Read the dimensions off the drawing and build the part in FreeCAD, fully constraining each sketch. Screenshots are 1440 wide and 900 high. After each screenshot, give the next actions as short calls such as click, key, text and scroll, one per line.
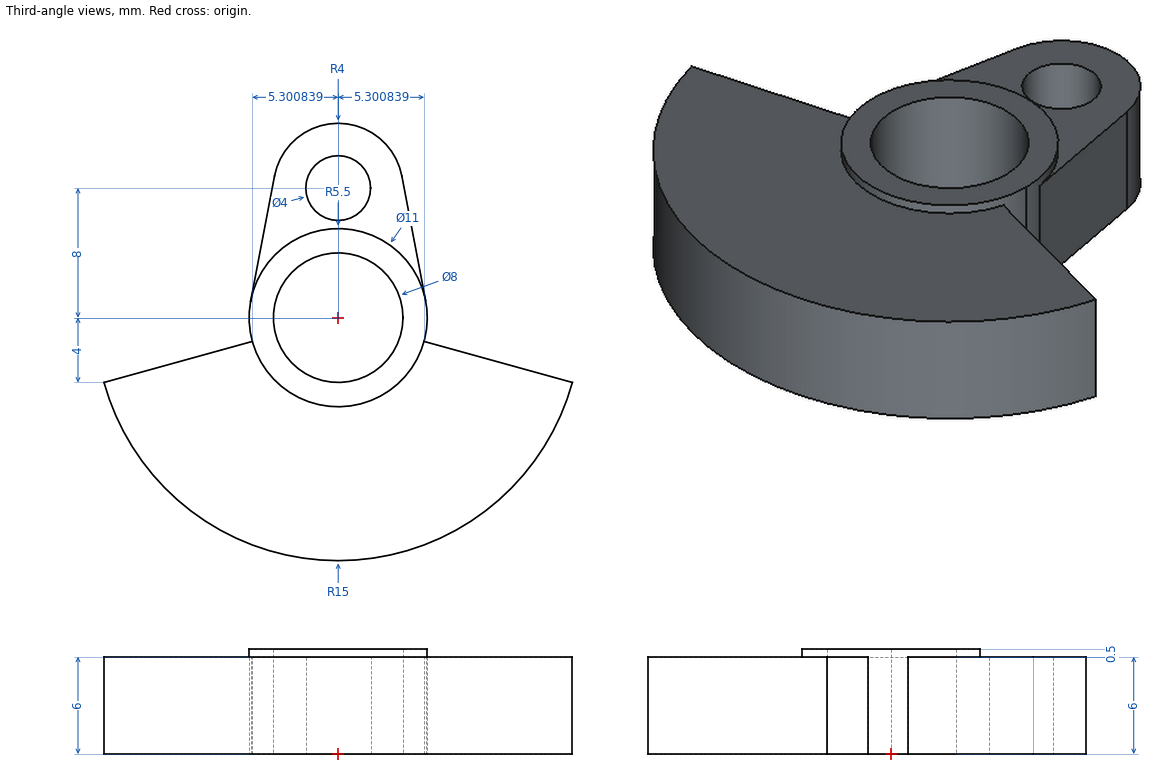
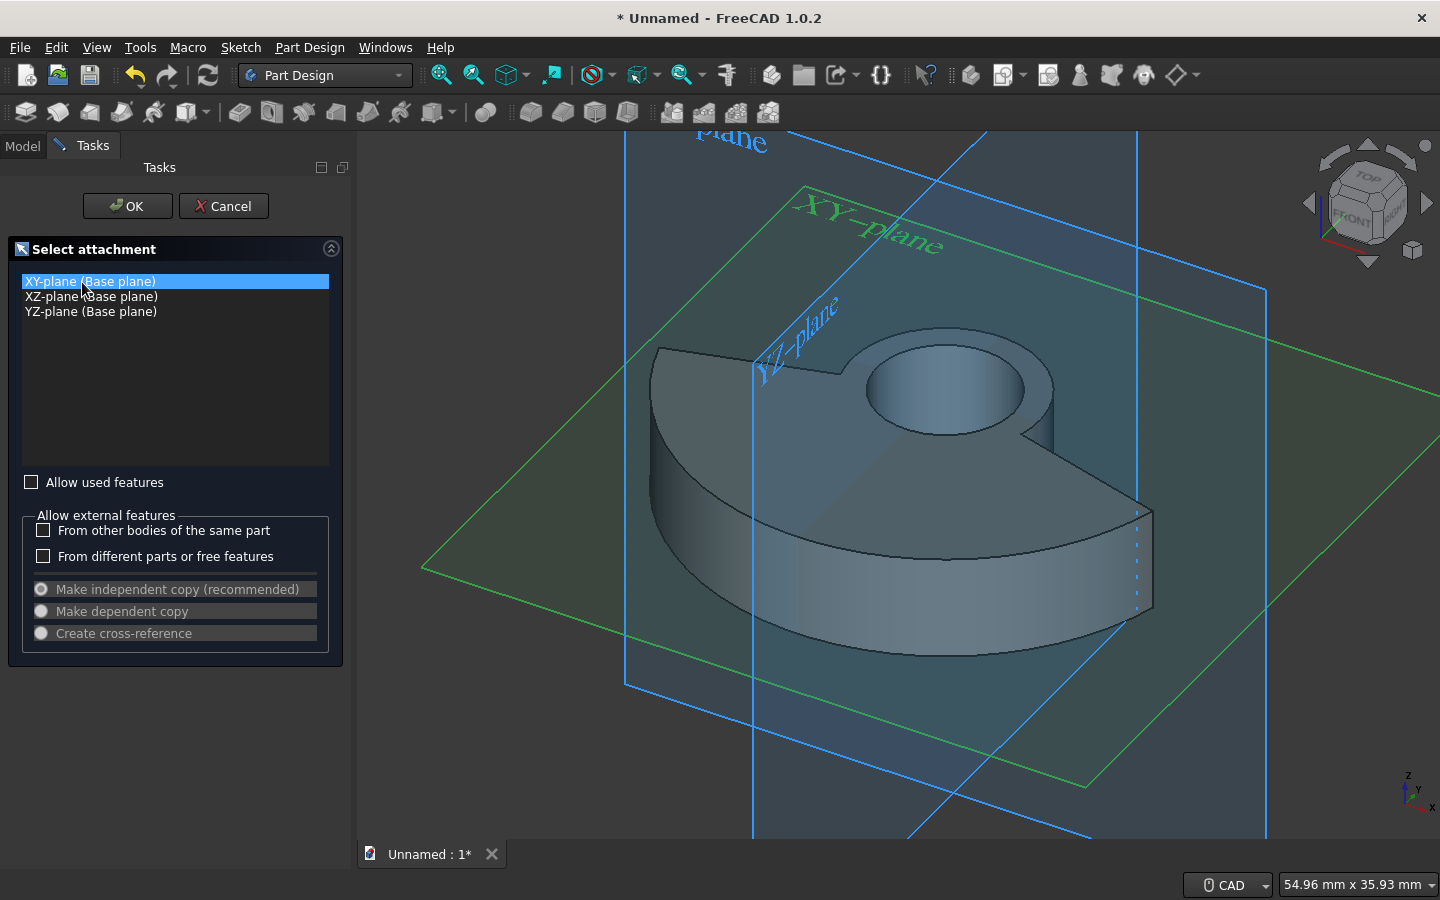
click(128, 206)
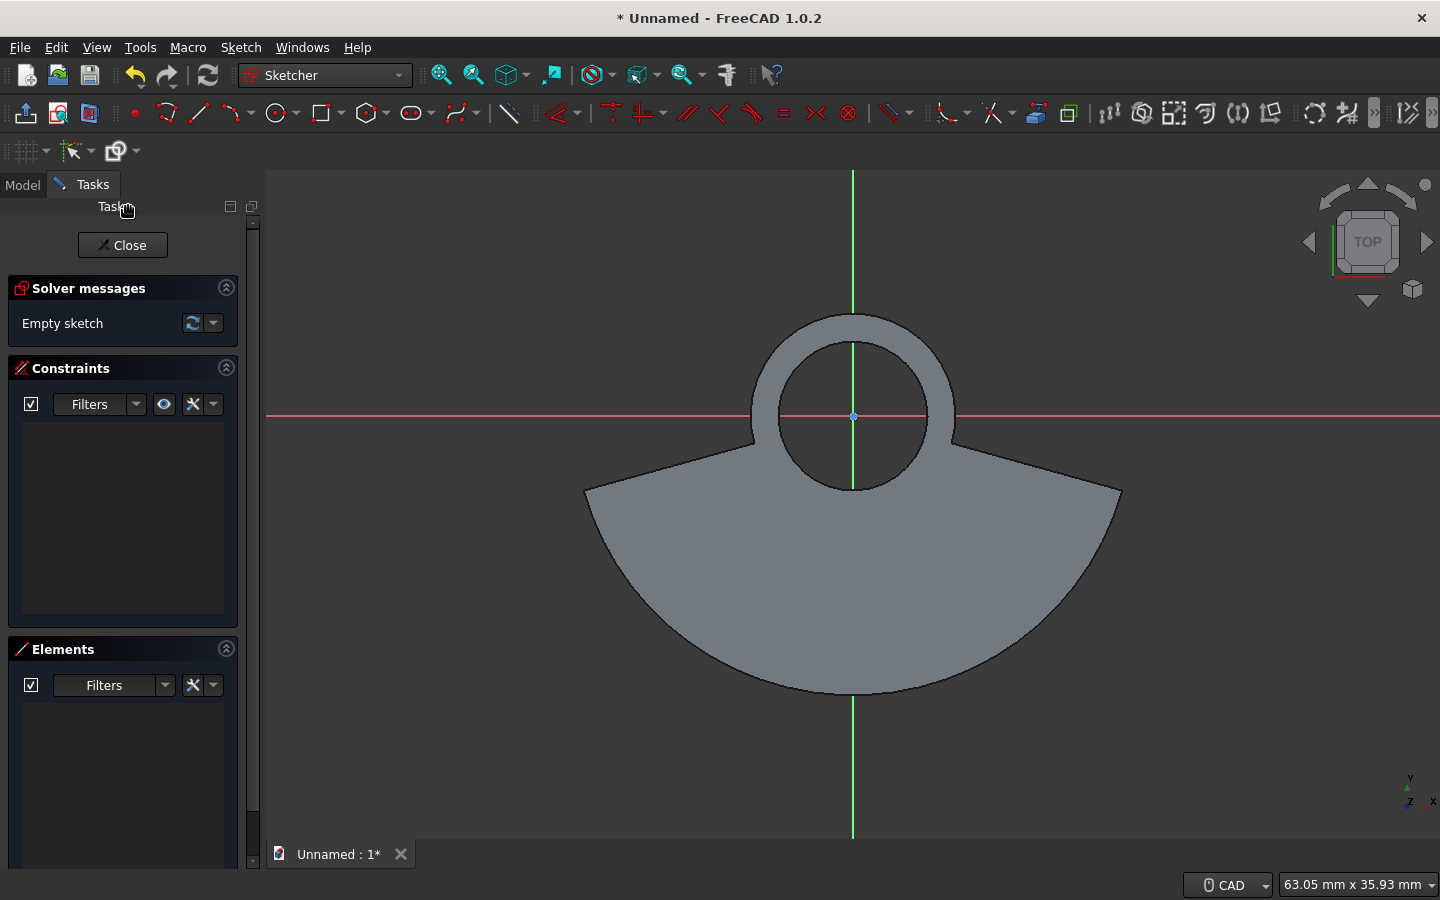
key(q)
key(s)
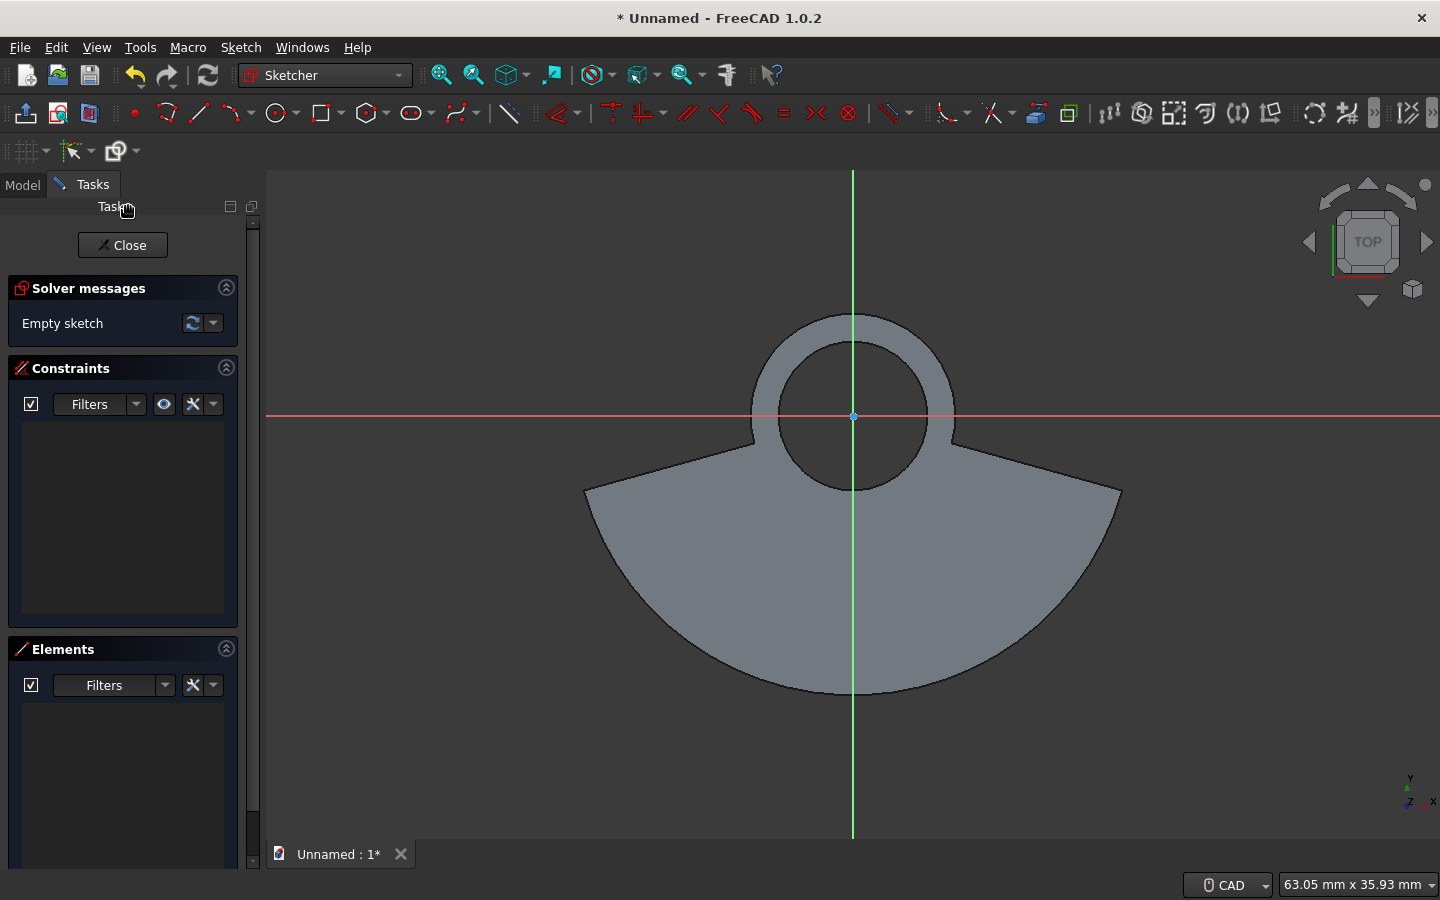
scroll(784, 504, down, 5)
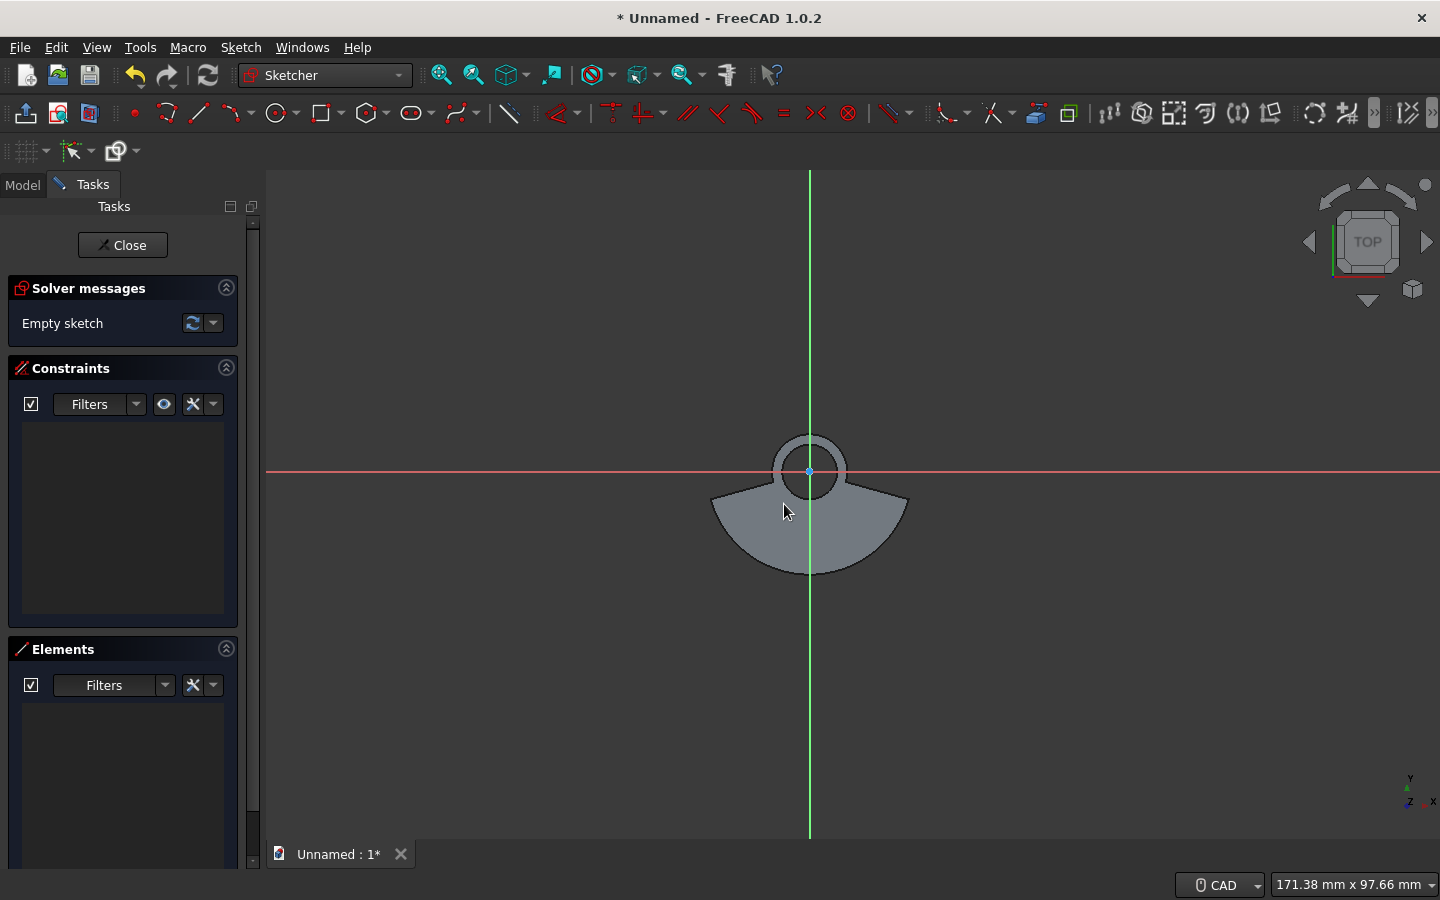
scroll(816, 412, up, 8)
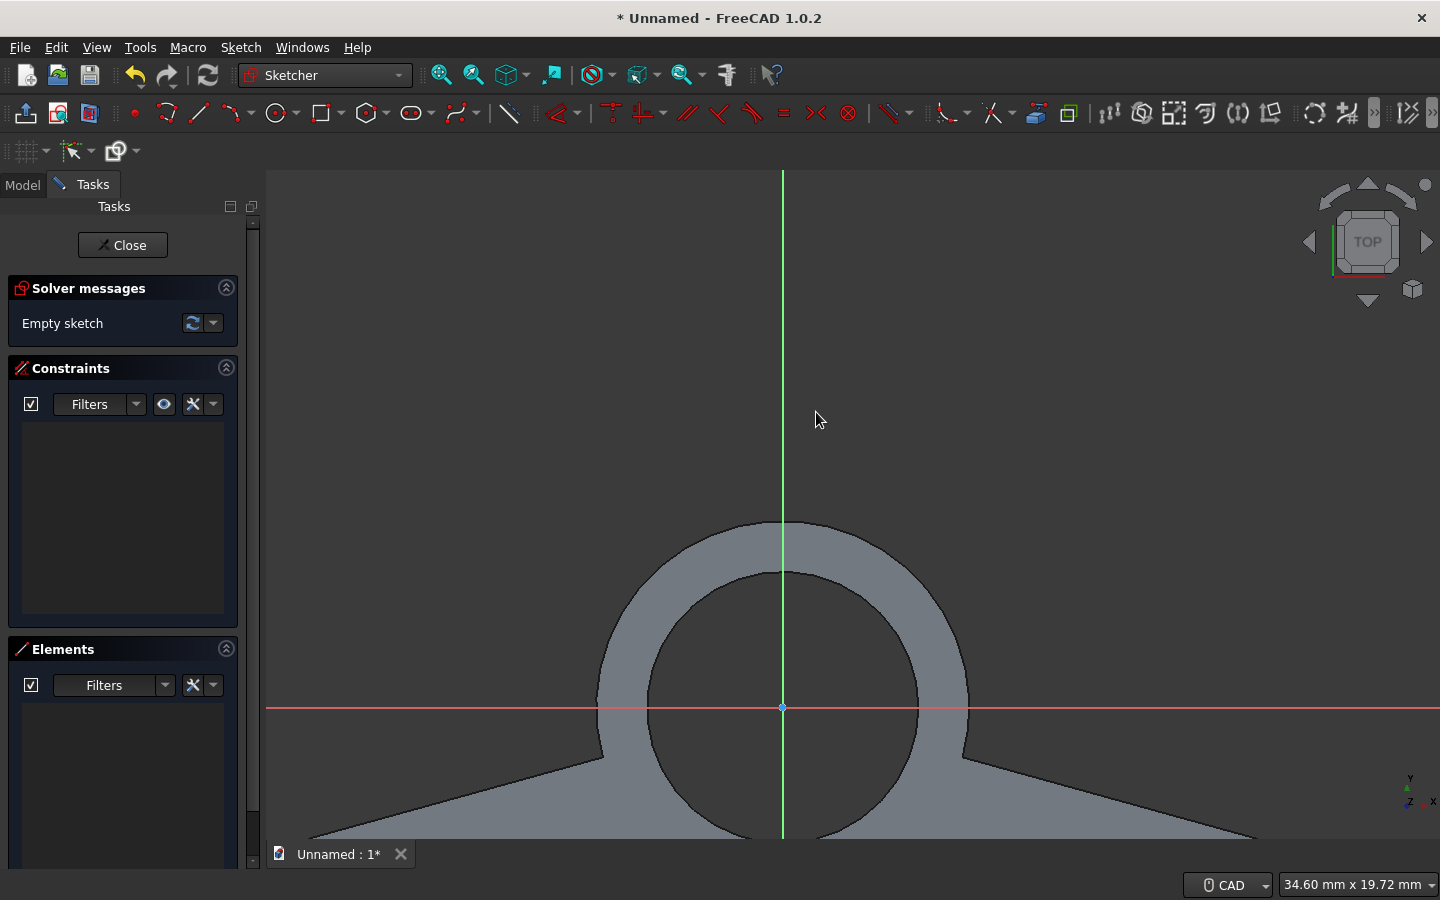
click(200, 114)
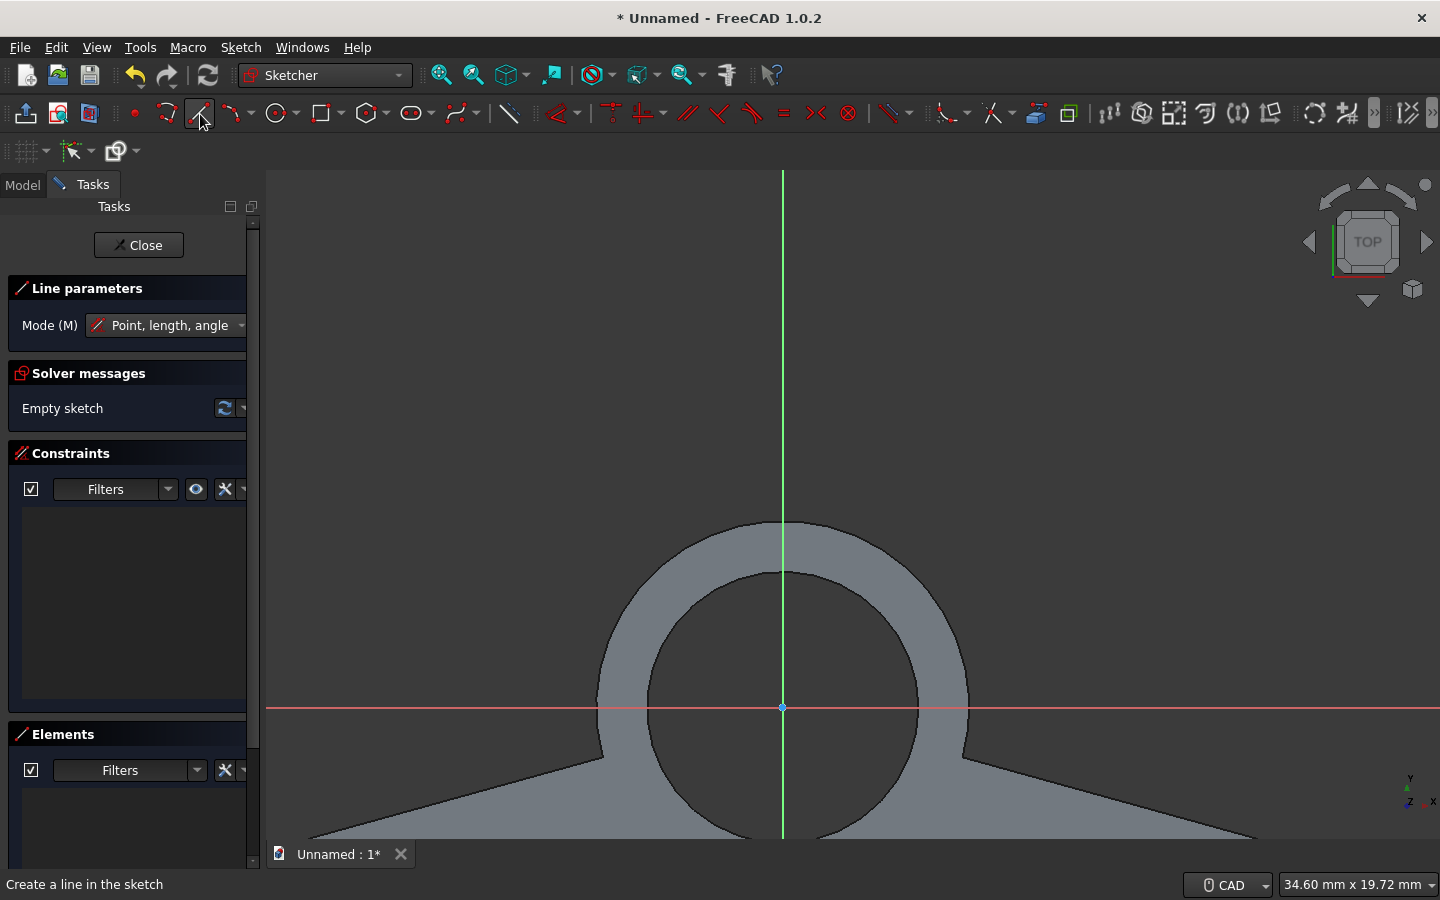
click(649, 411)
click(599, 673)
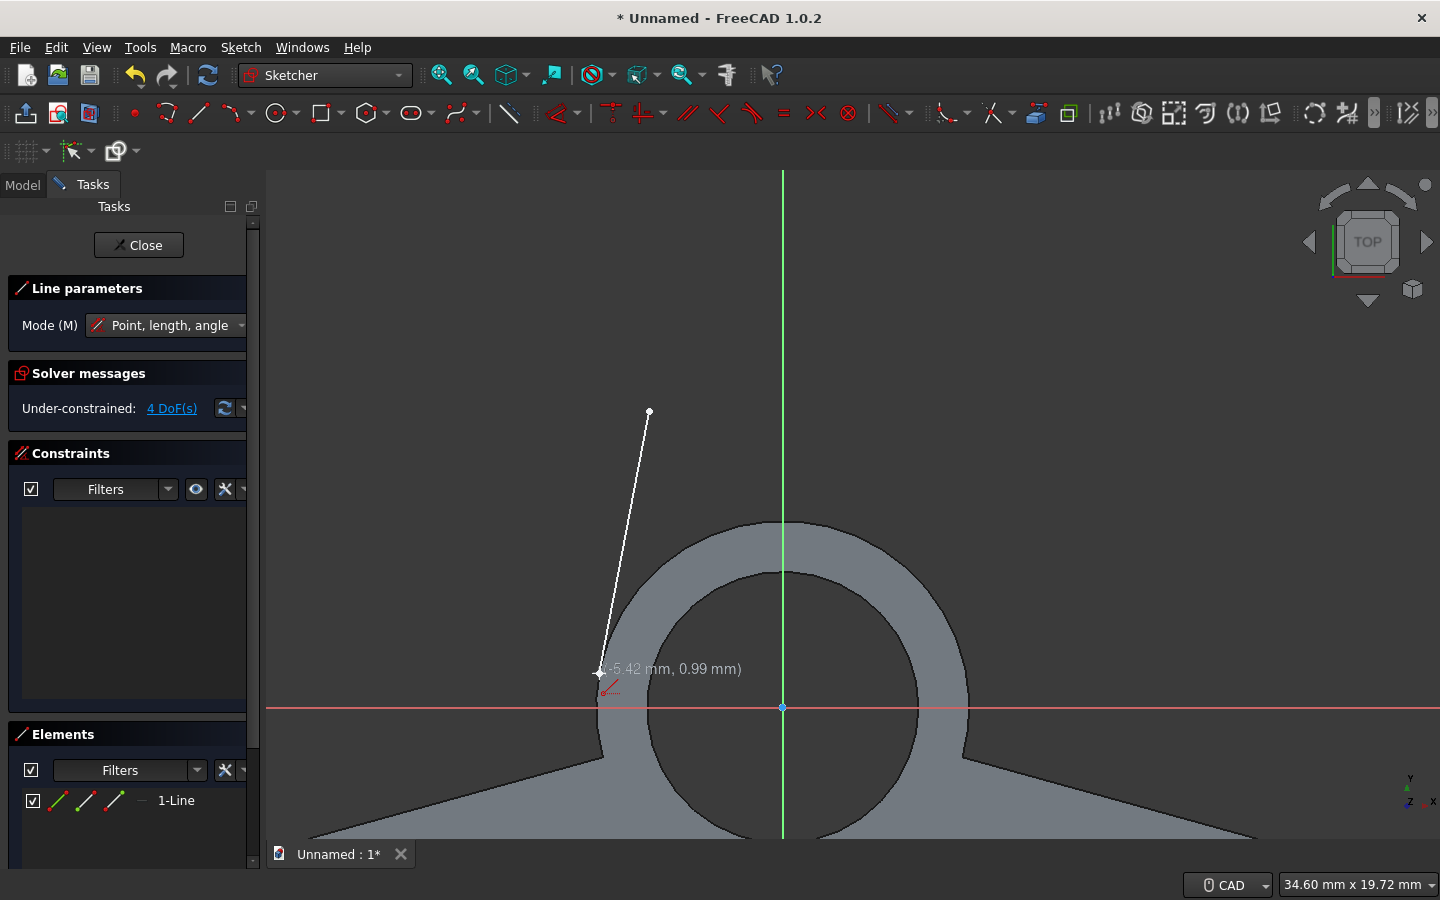
click(966, 673)
click(916, 411)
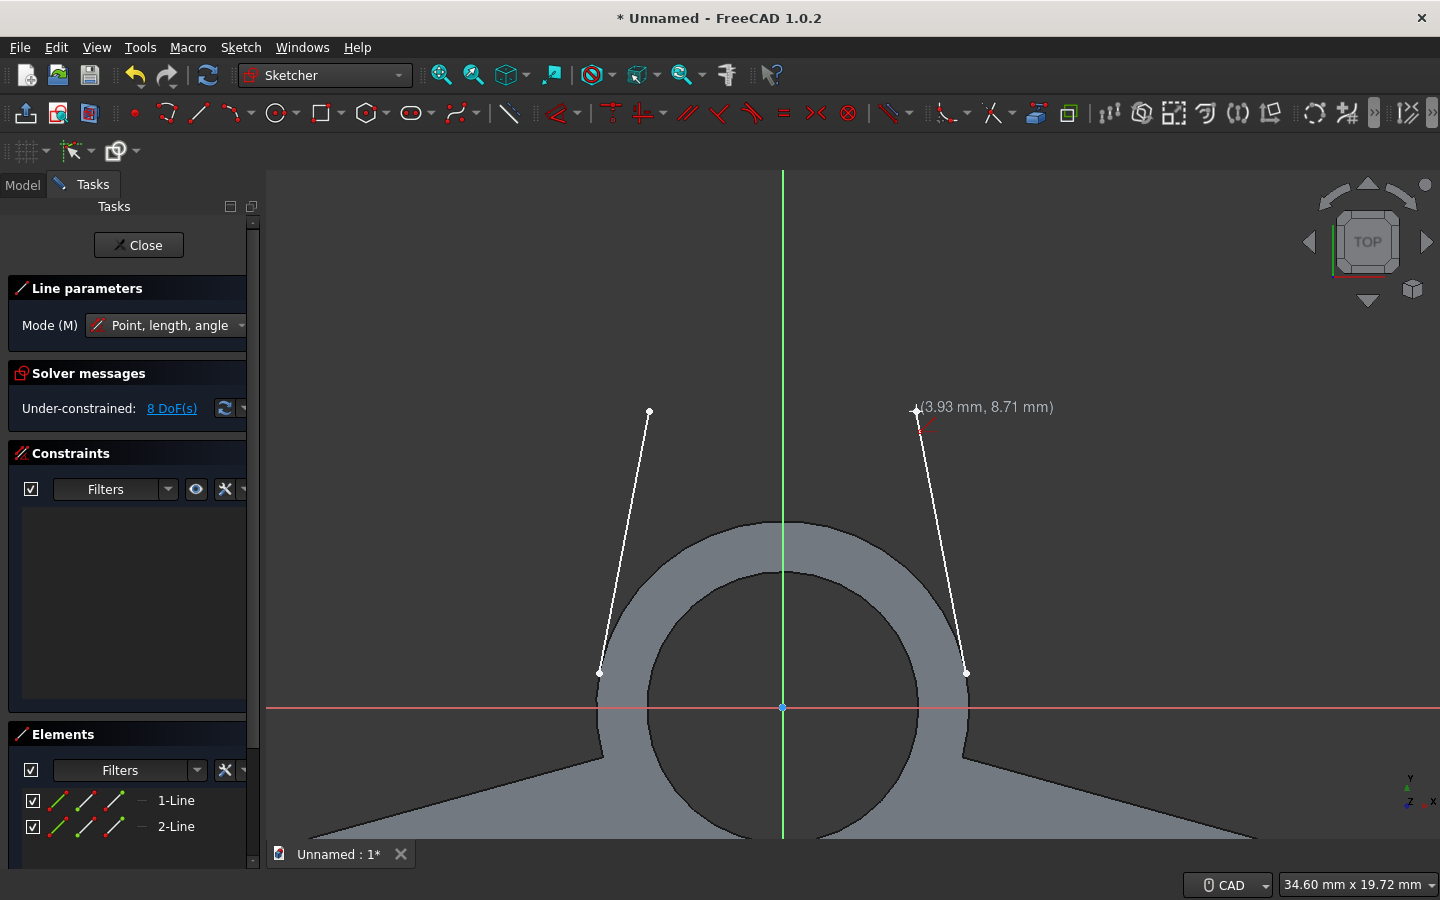
click(232, 114)